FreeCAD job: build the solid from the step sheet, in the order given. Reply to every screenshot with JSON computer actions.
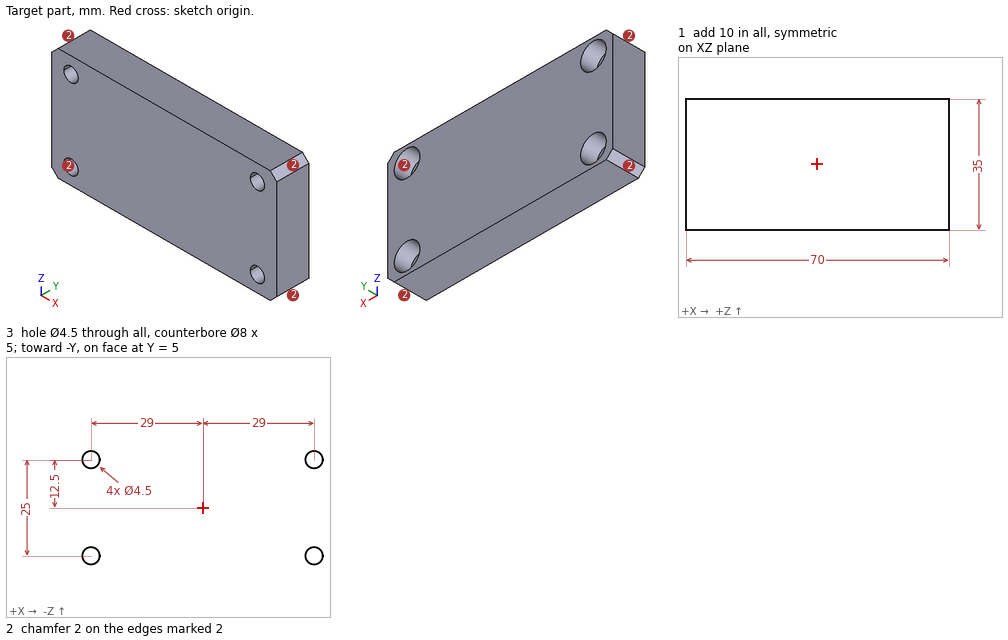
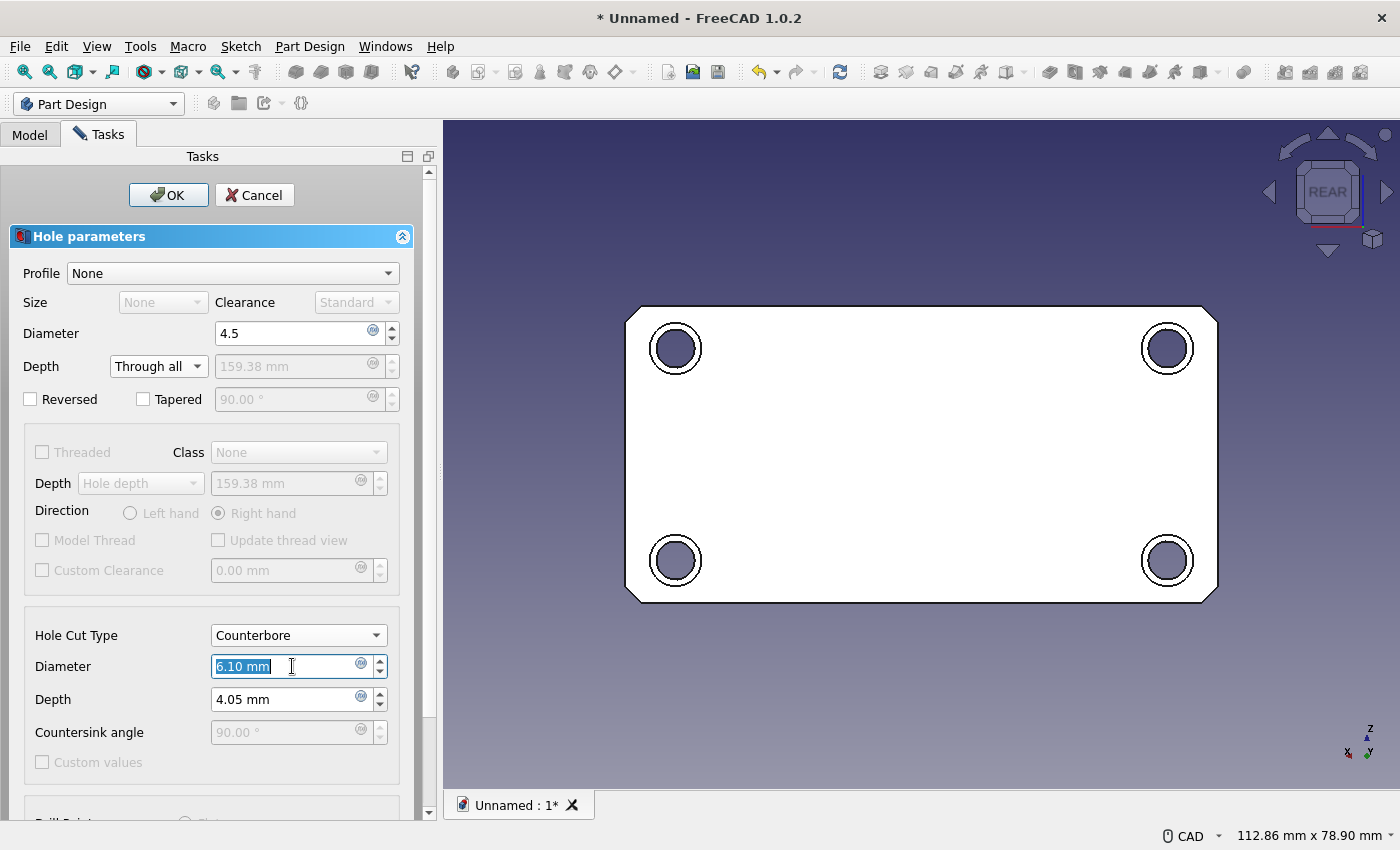
{"action": "type", "text": "8"}
{"action": "key", "text": "Tab"}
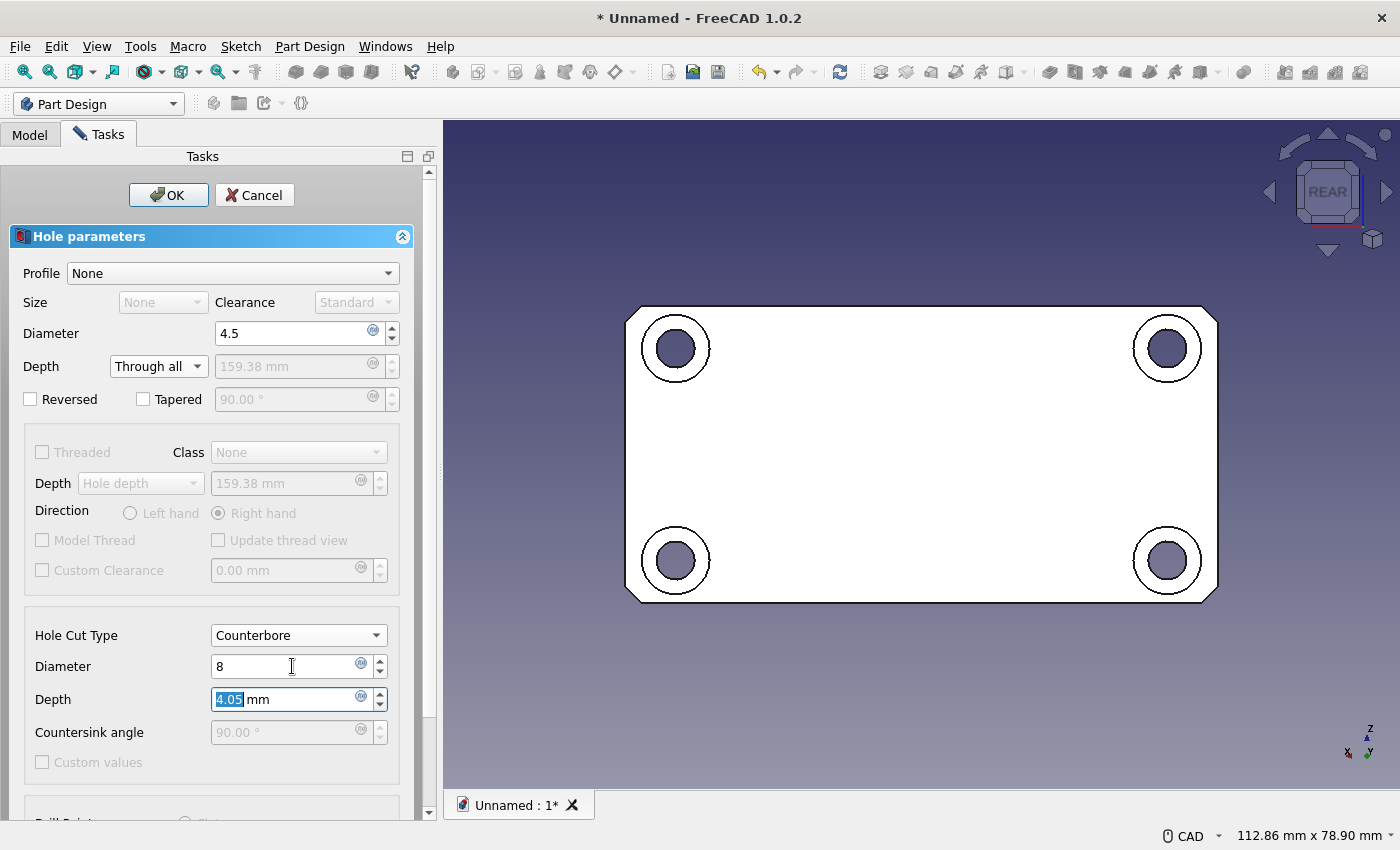
{"action": "type", "text": "5"}
{"action": "key", "text": "Tab"}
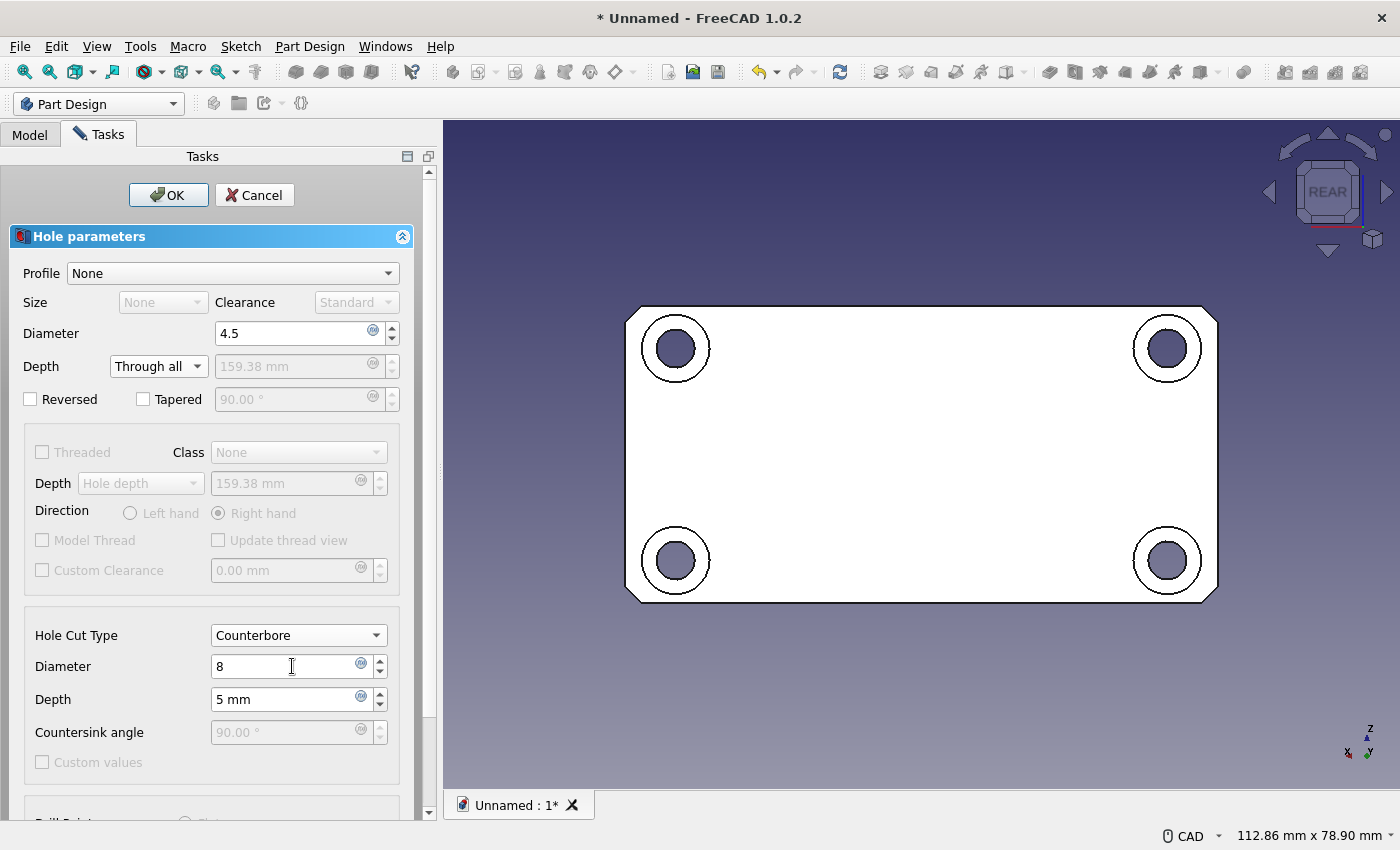
{"action": "left_click", "coordinate": [169, 195]}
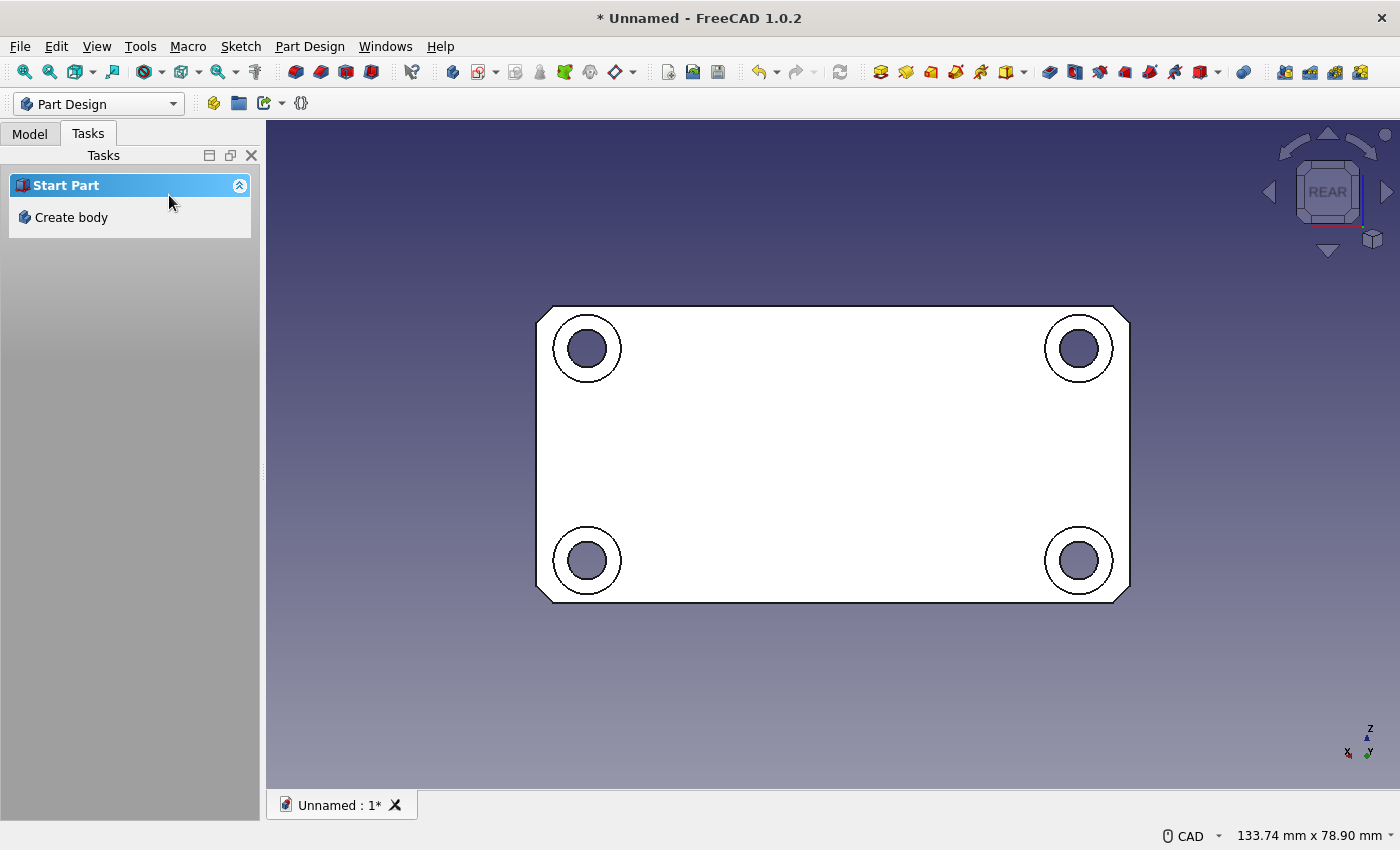
{"action": "key", "text": "0"}